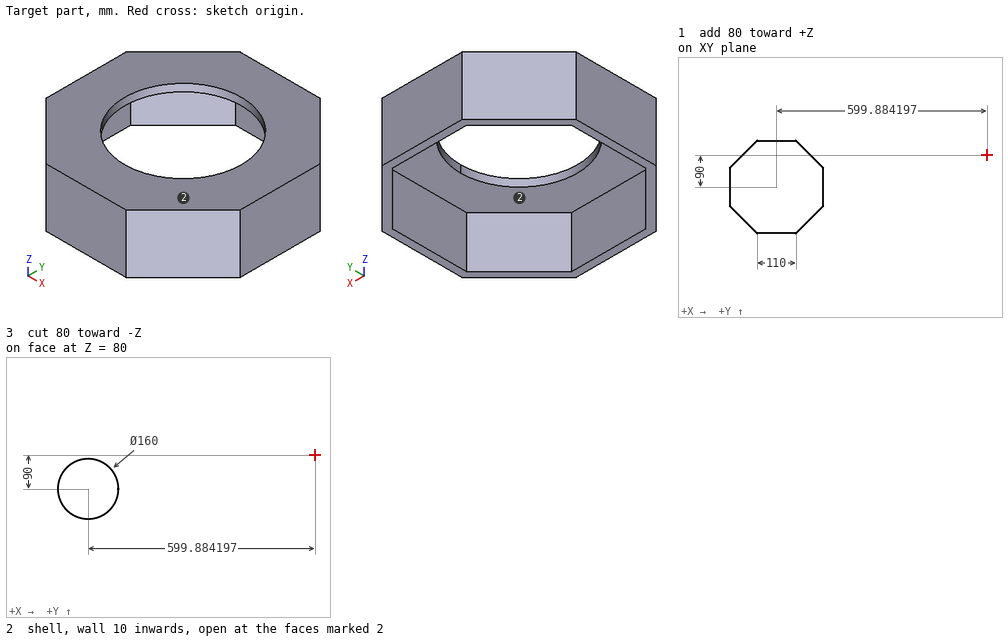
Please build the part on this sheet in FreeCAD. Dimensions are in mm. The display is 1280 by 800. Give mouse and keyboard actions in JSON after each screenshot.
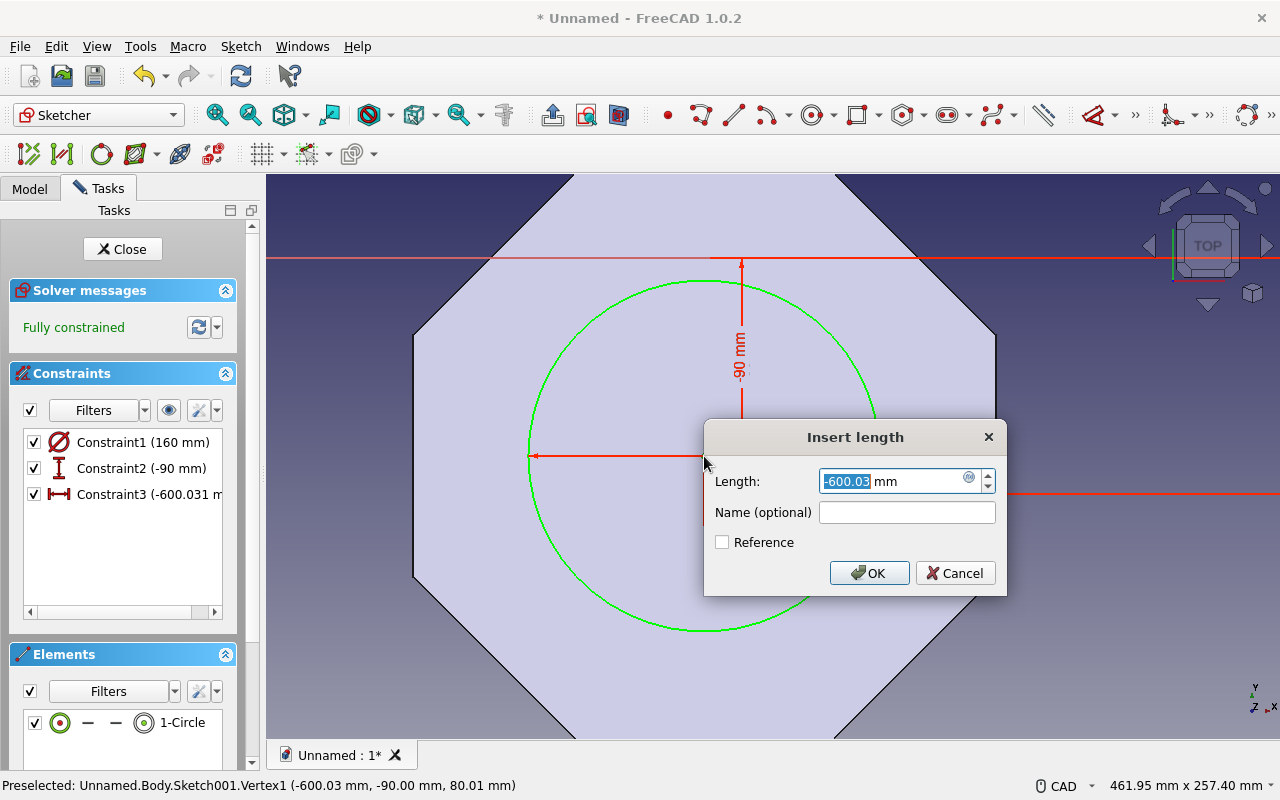
{"action": "type", "text": "-599.884197"}
{"action": "key", "text": "Return"}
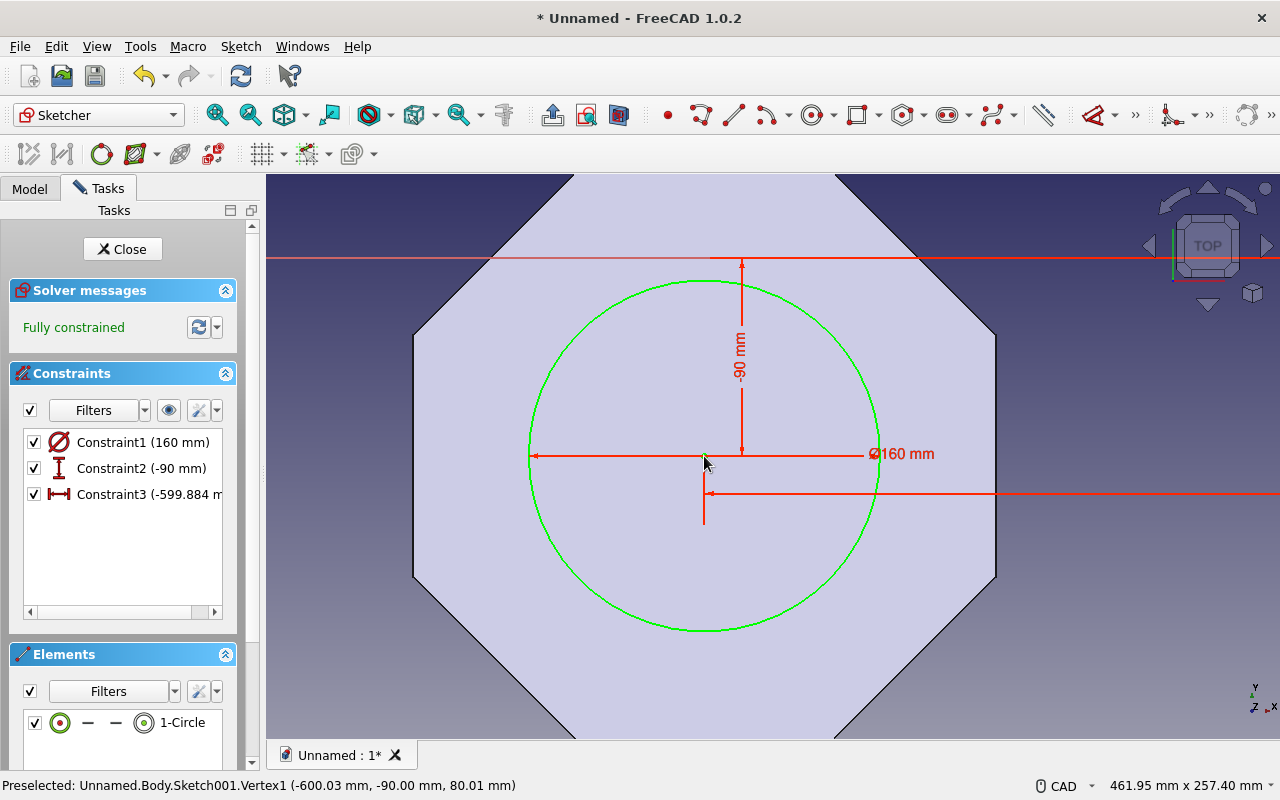
{"action": "left_click", "coordinate": [123, 249]}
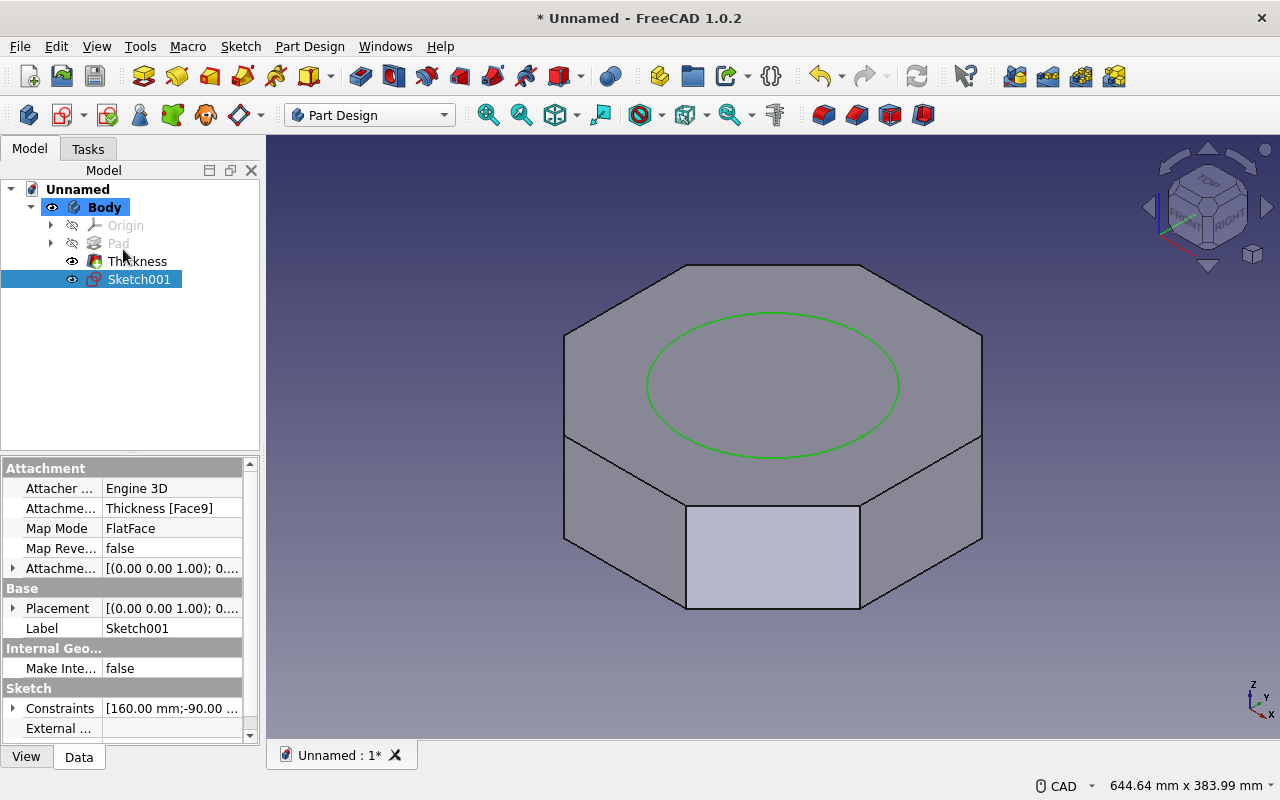
{"action": "left_click", "coordinate": [361, 76]}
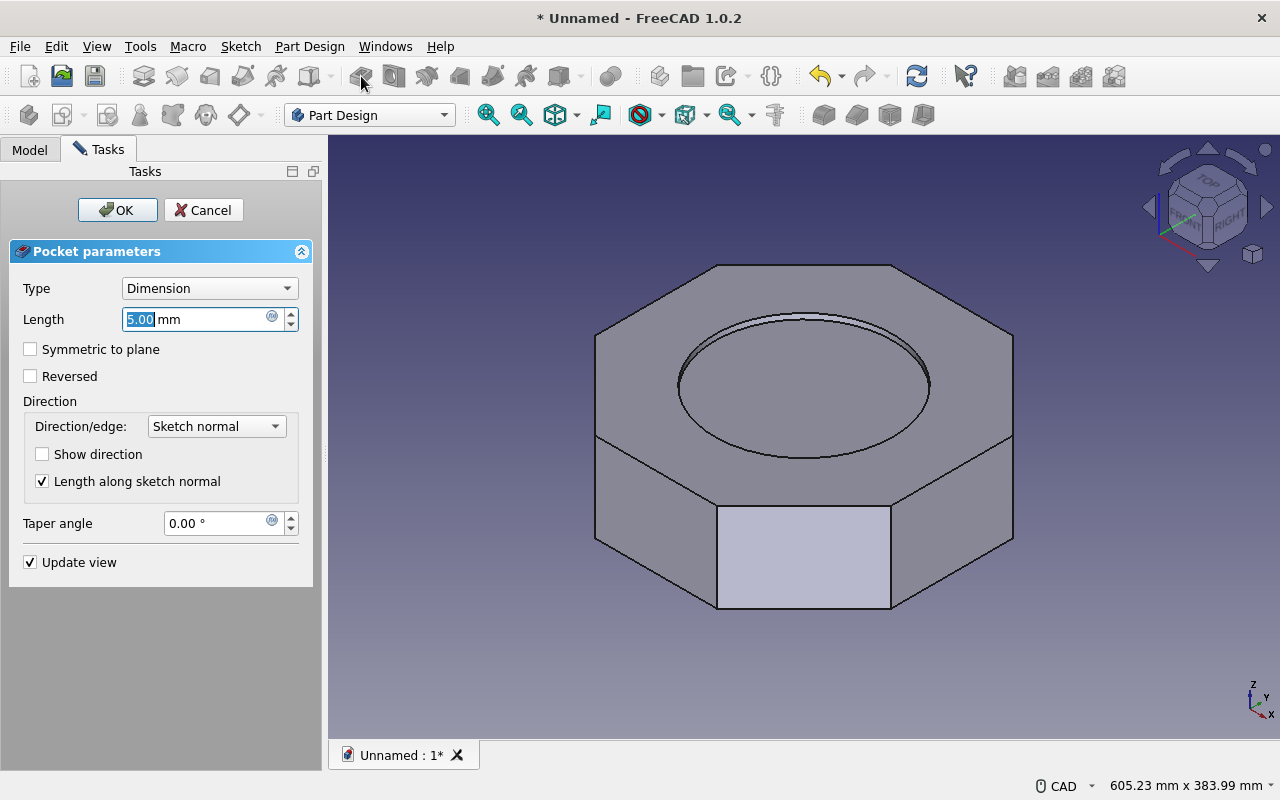
{"action": "type", "text": "80"}
{"action": "key", "text": "Tab"}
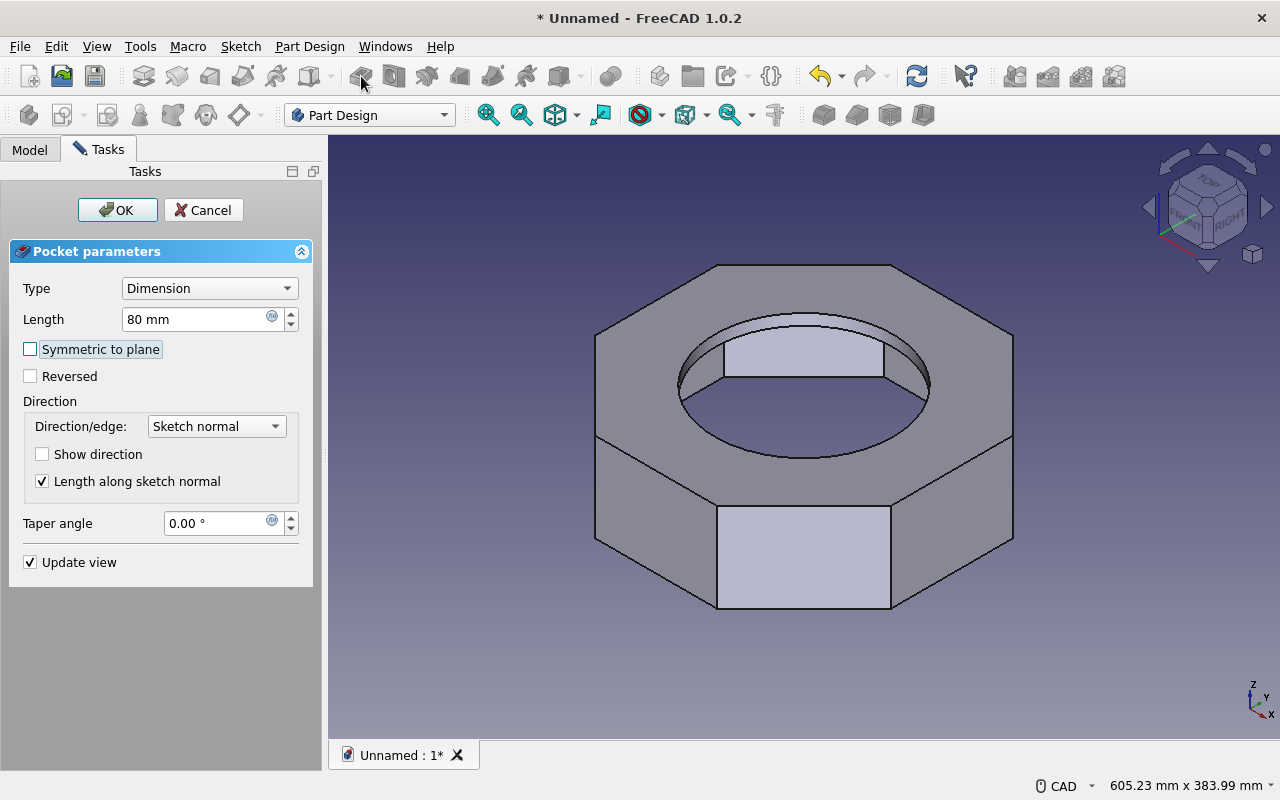
{"action": "left_click", "coordinate": [118, 210]}